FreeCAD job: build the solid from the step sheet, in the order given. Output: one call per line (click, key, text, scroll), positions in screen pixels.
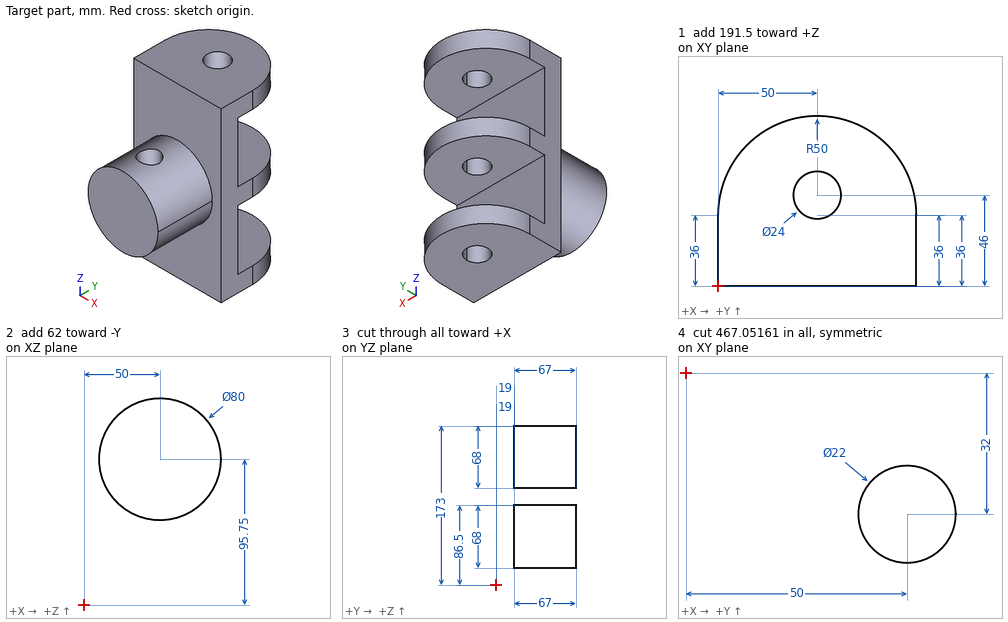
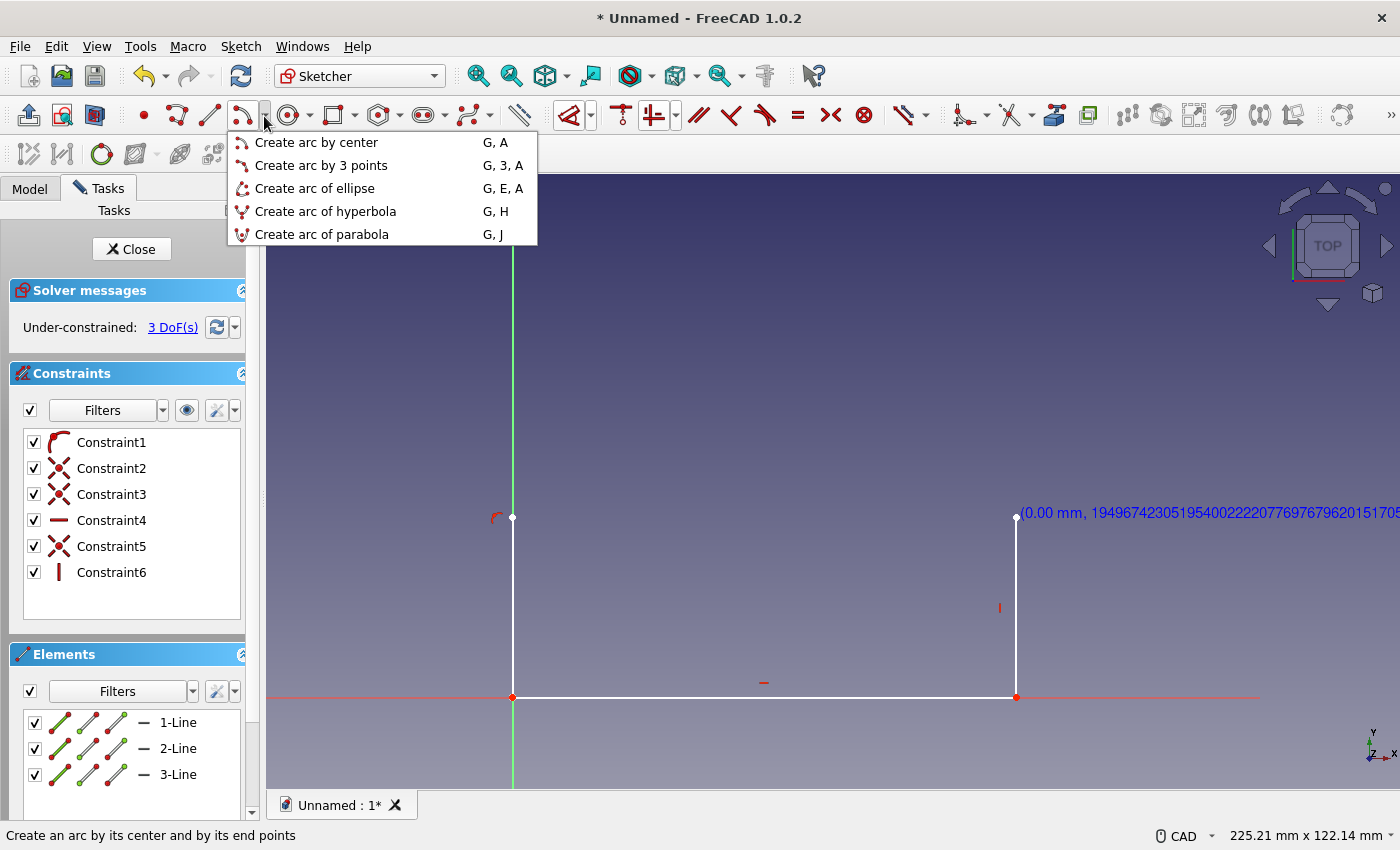
click(382, 166)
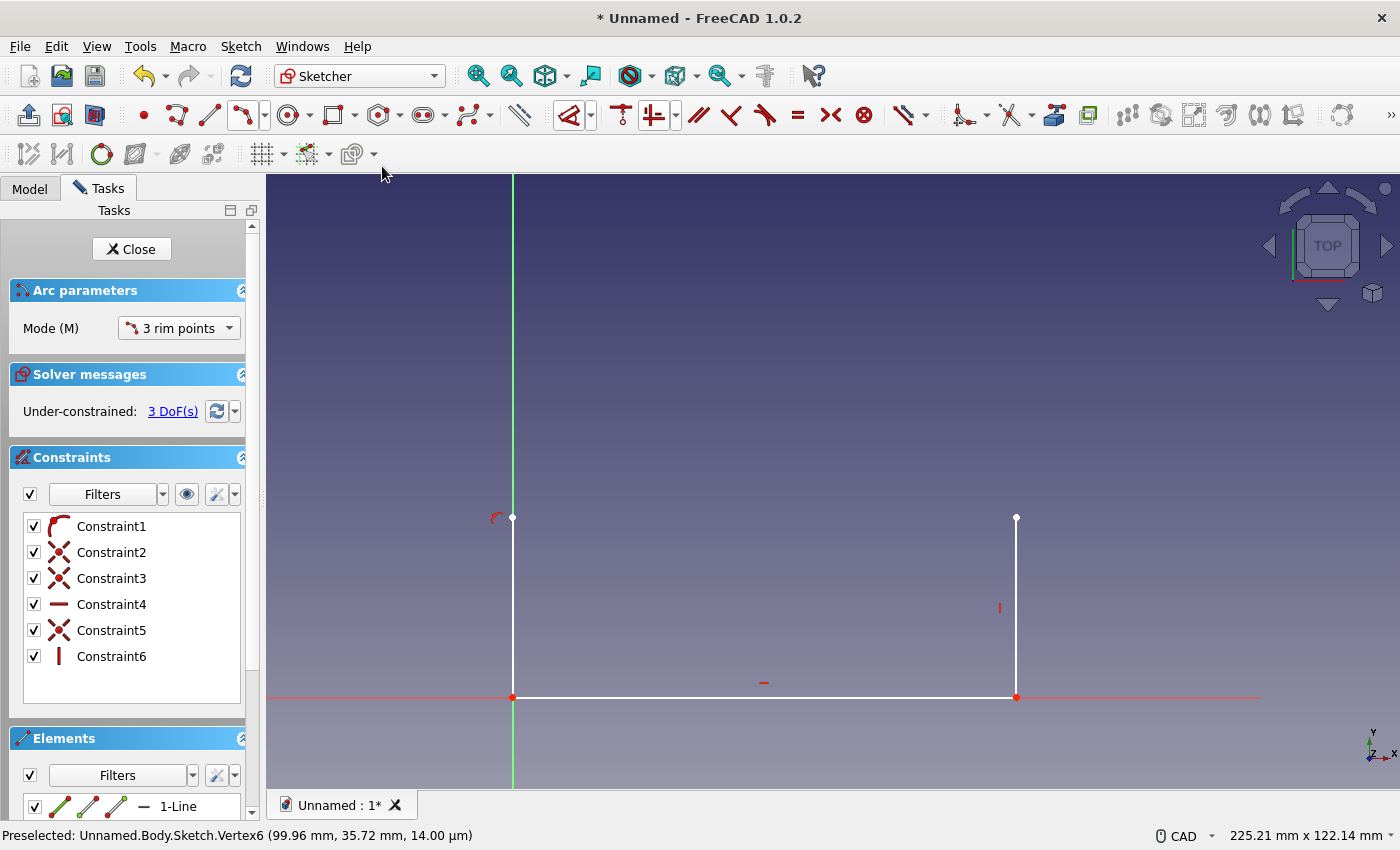
click(1016, 518)
click(513, 518)
click(764, 265)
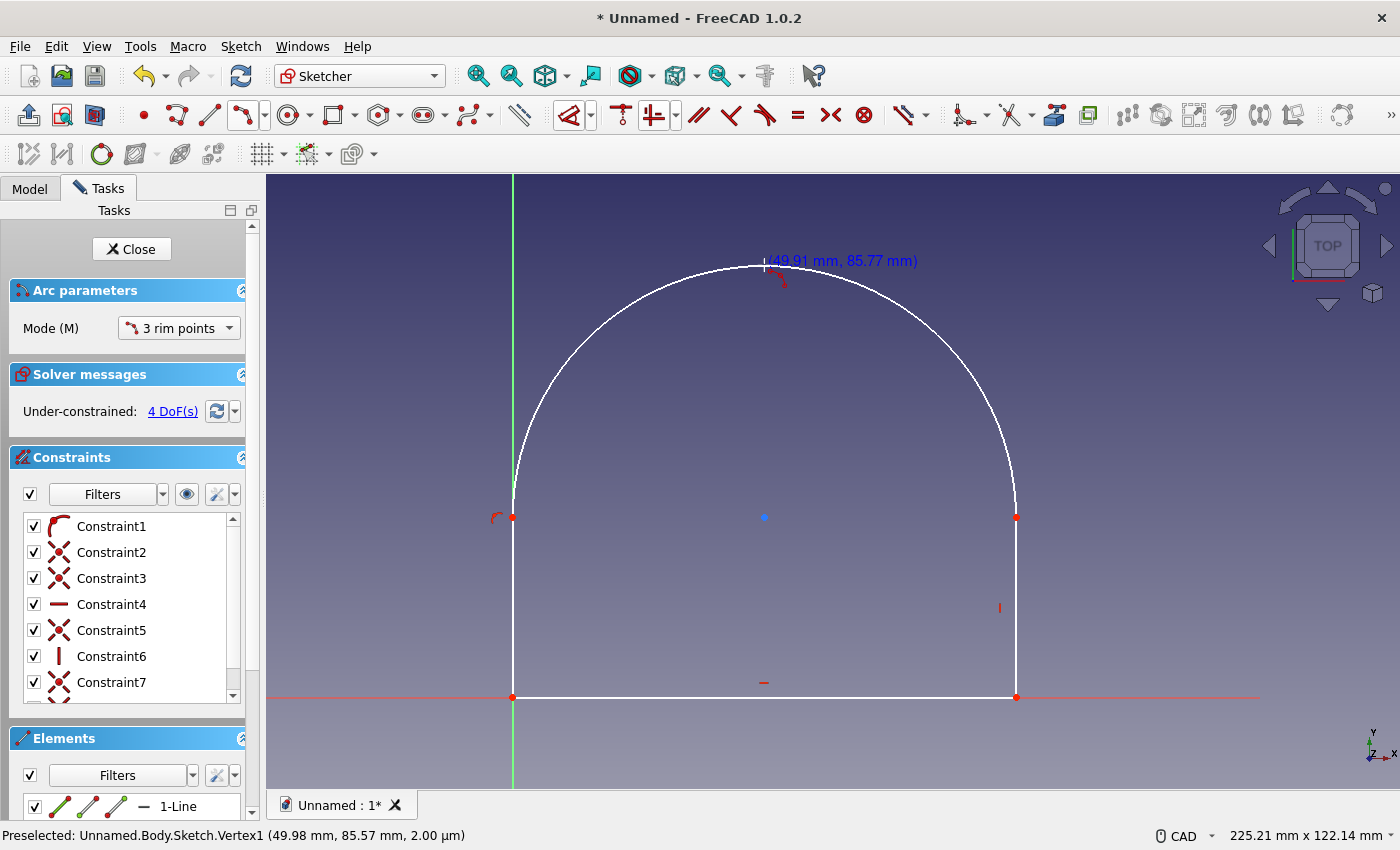
click(288, 116)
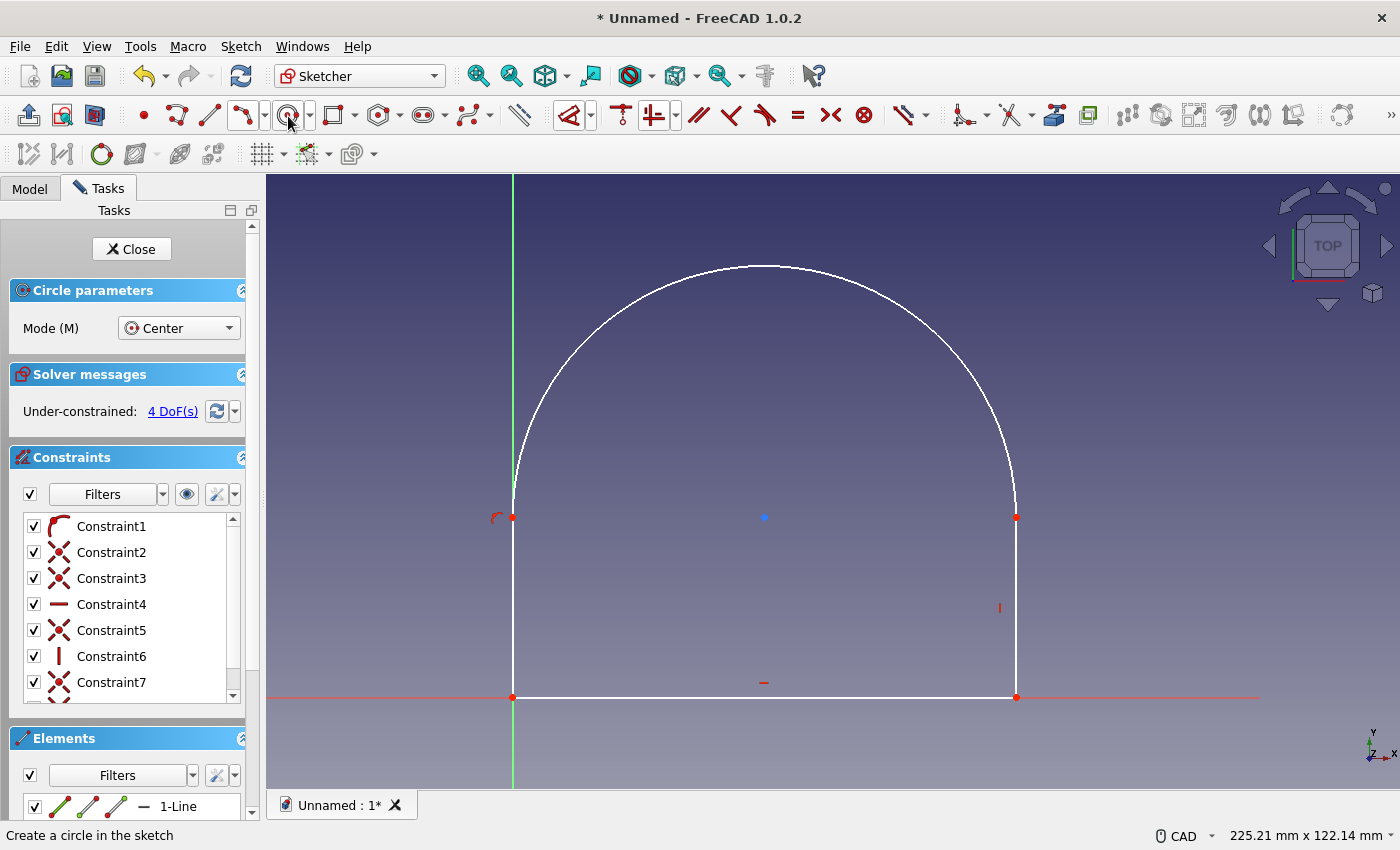
click(764, 466)
click(807, 424)
key(Escape)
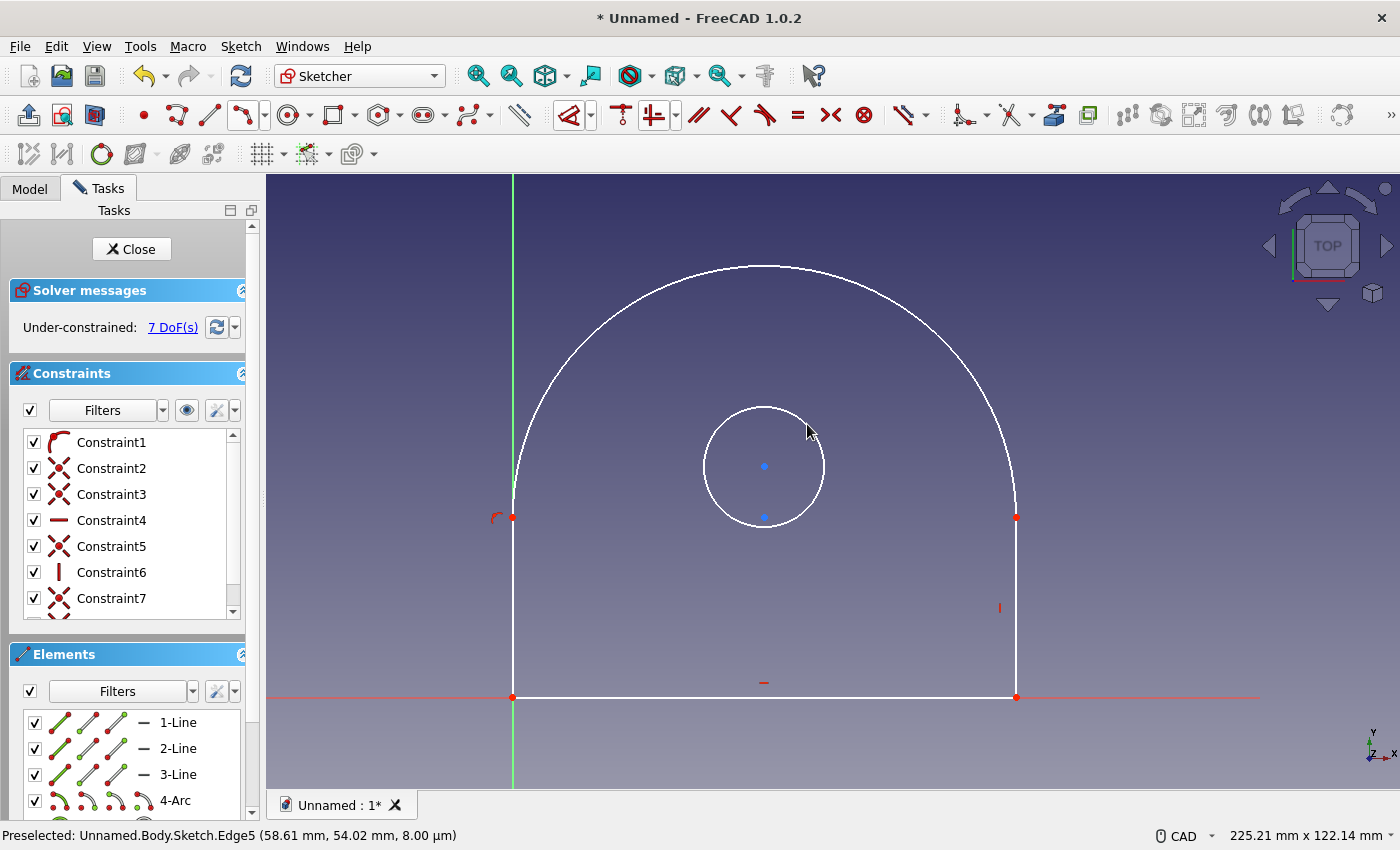
click(568, 116)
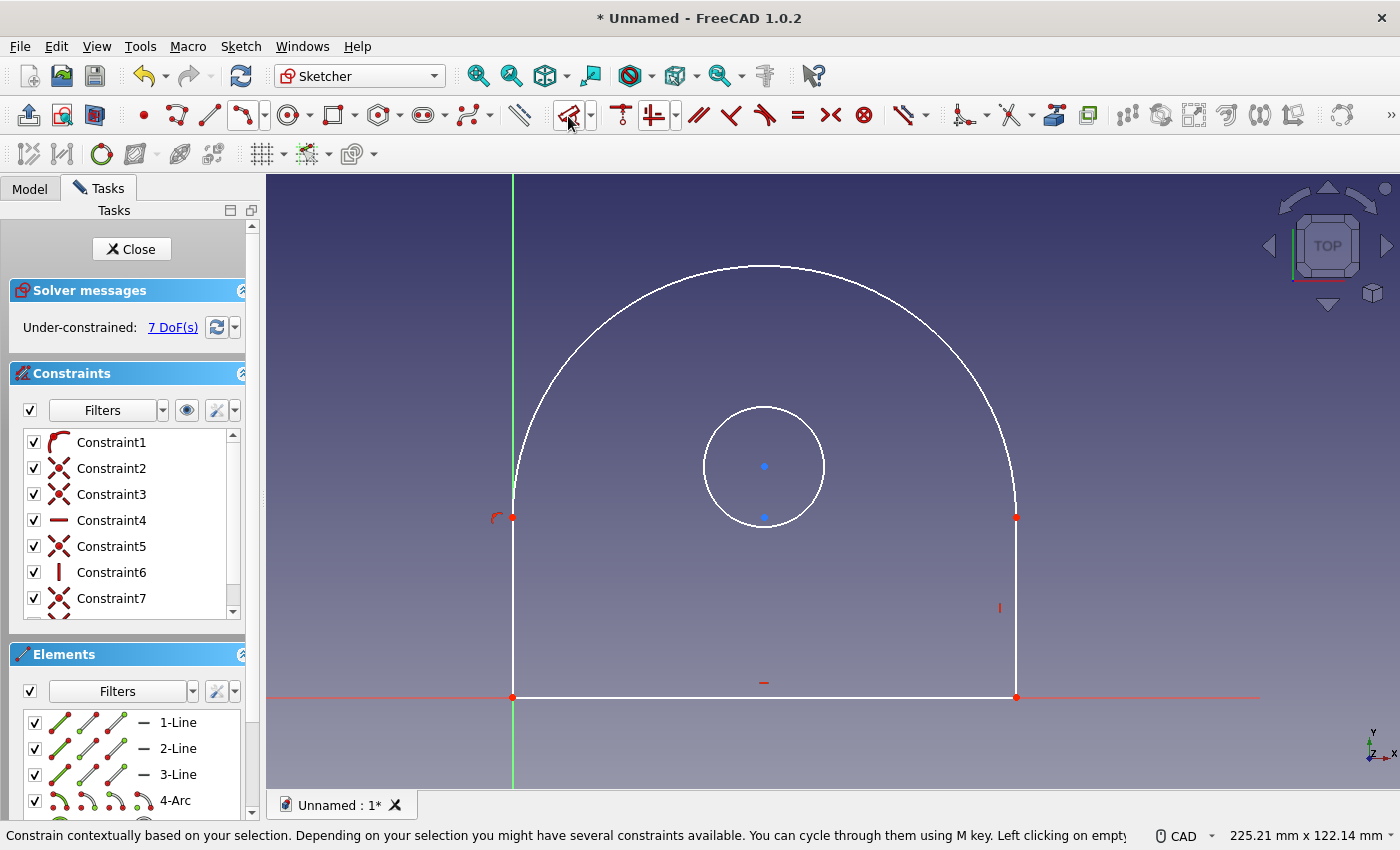
click(912, 314)
click(931, 288)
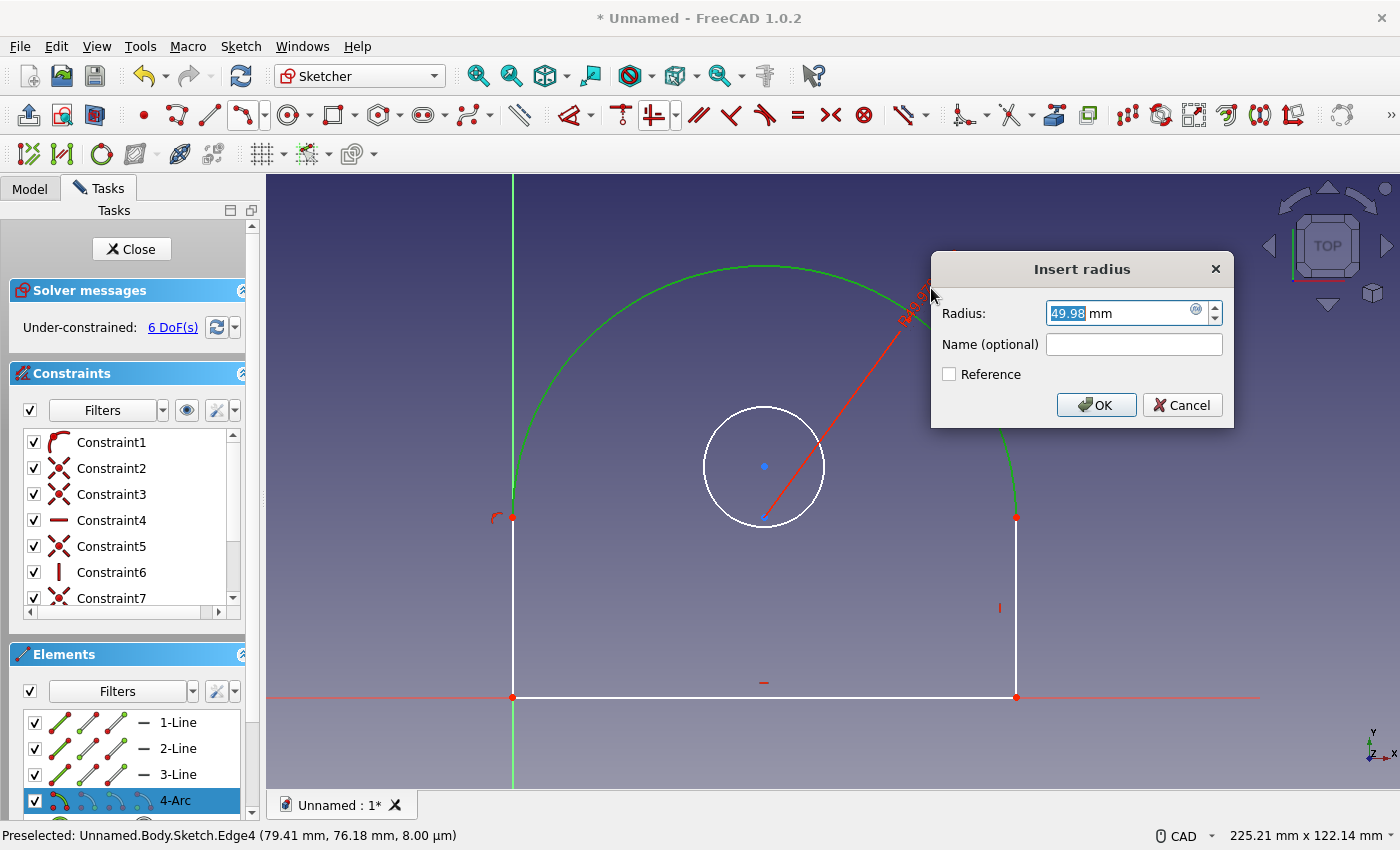
text(50)
key(Return)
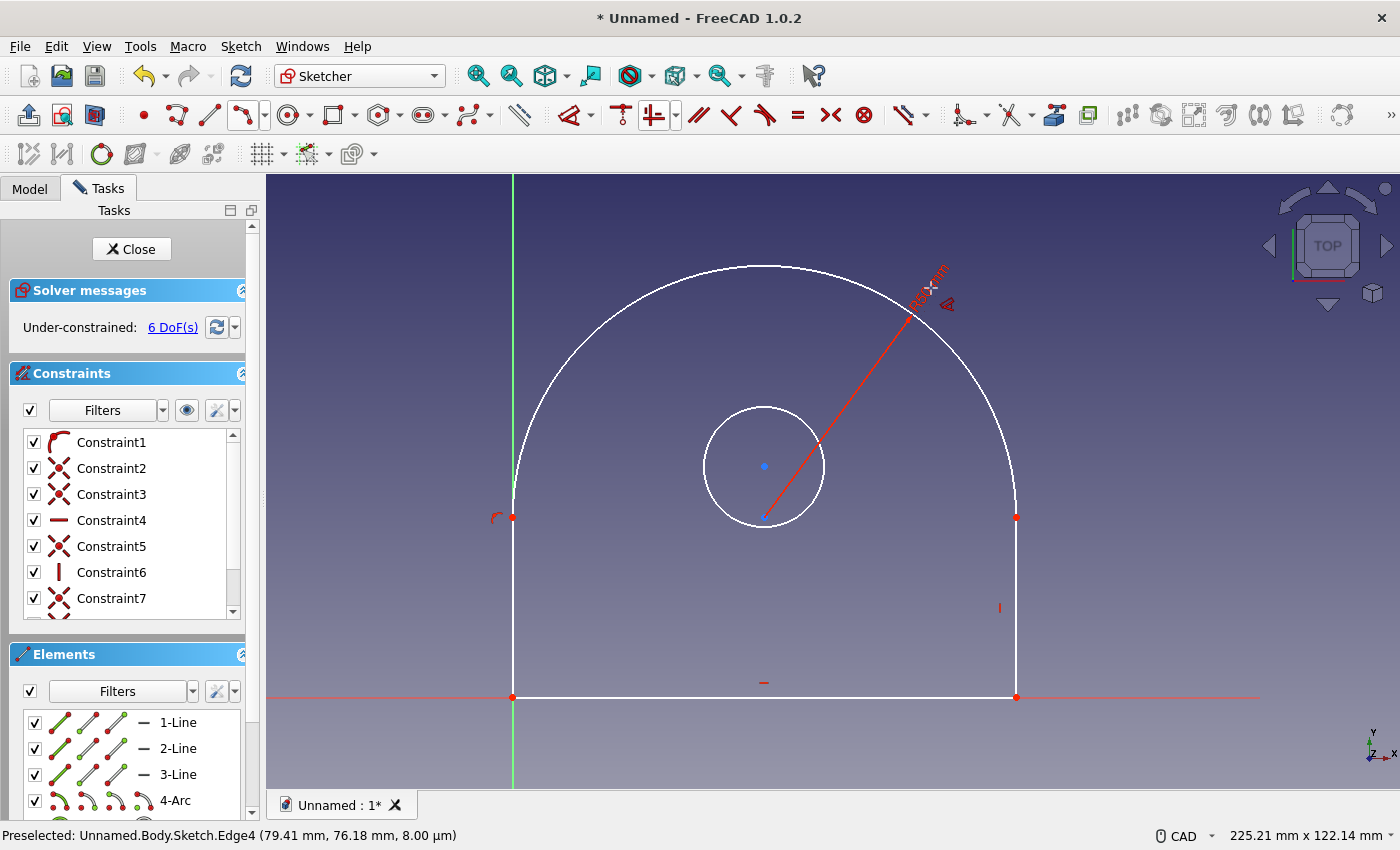
click(806, 424)
click(828, 401)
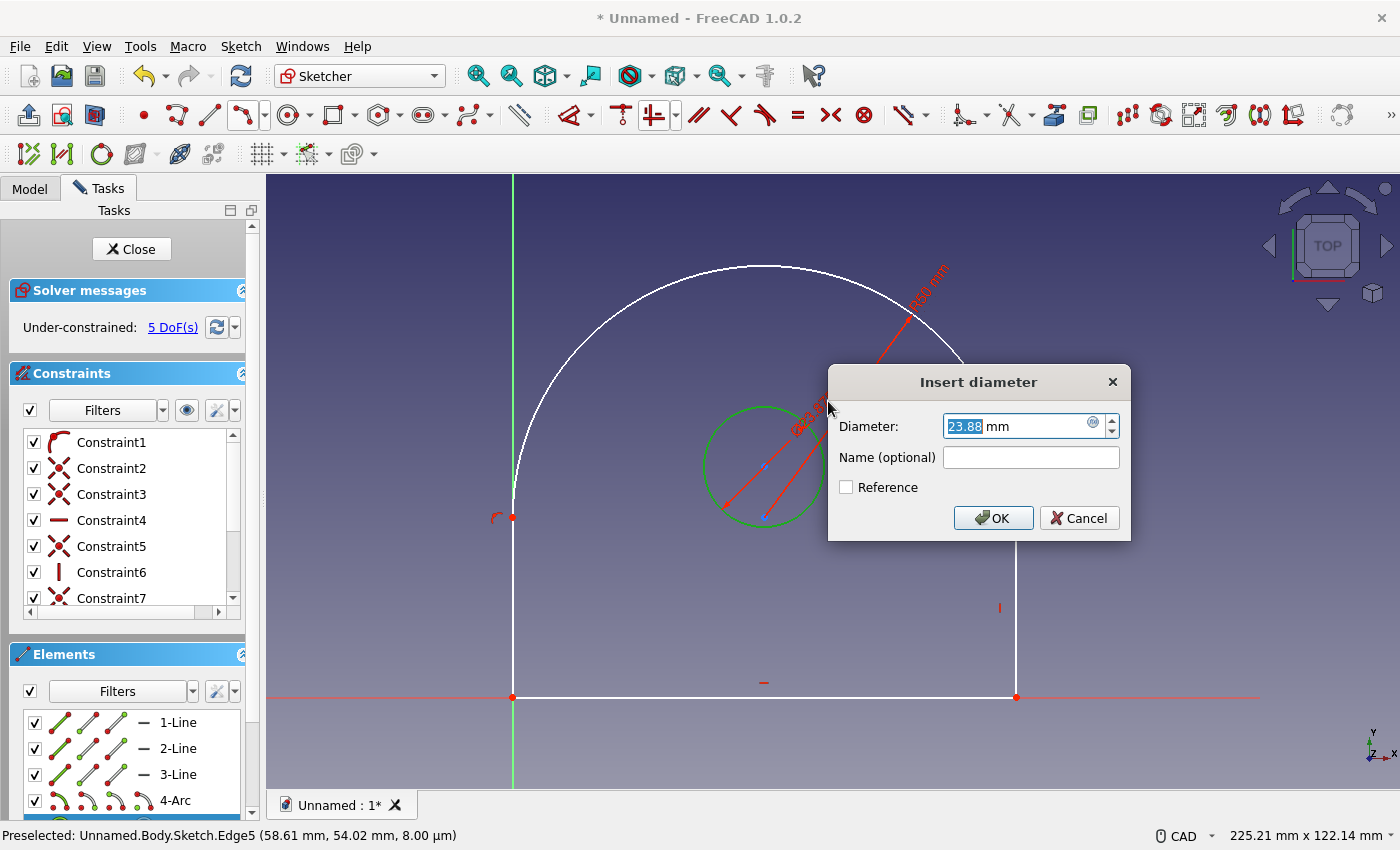
text(24)
key(Return)